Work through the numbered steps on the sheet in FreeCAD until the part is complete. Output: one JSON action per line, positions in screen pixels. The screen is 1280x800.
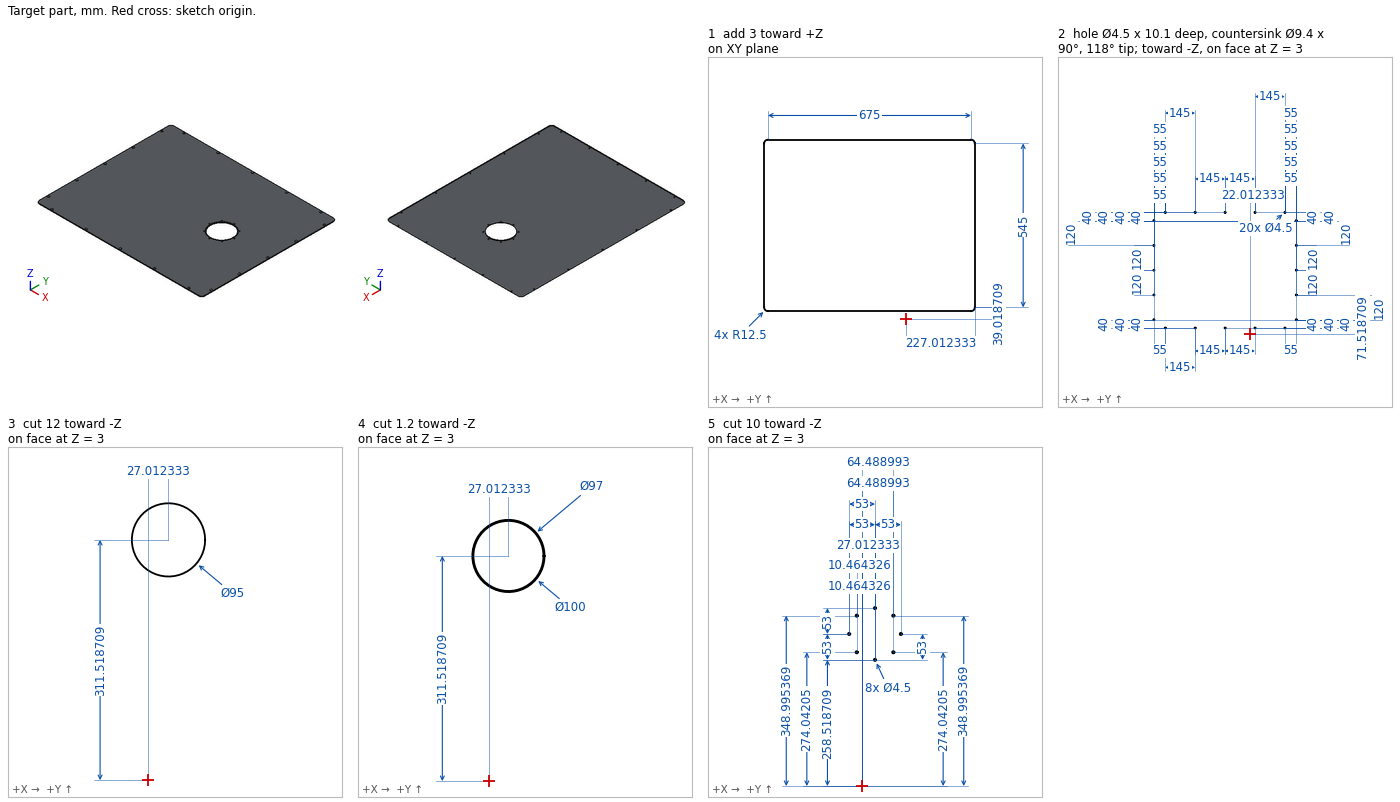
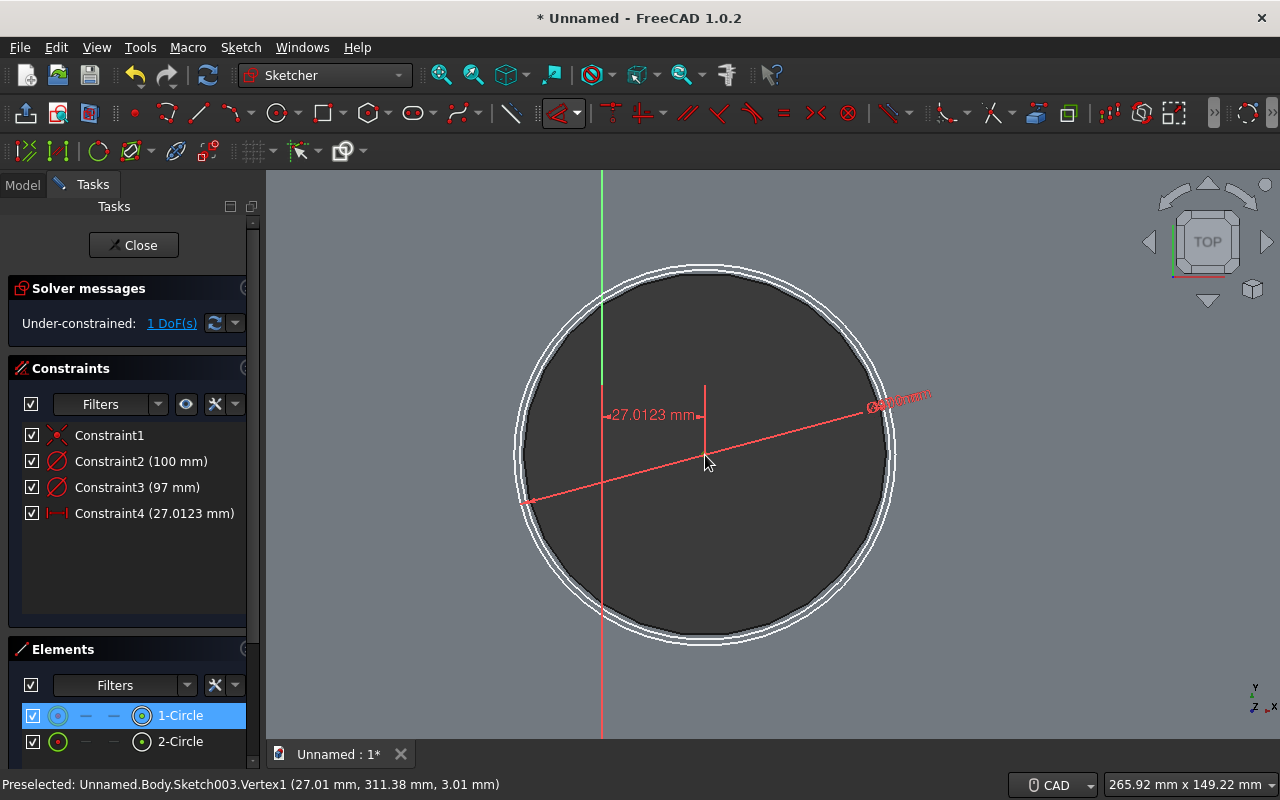
{"action": "left_click", "coordinate": [580, 114]}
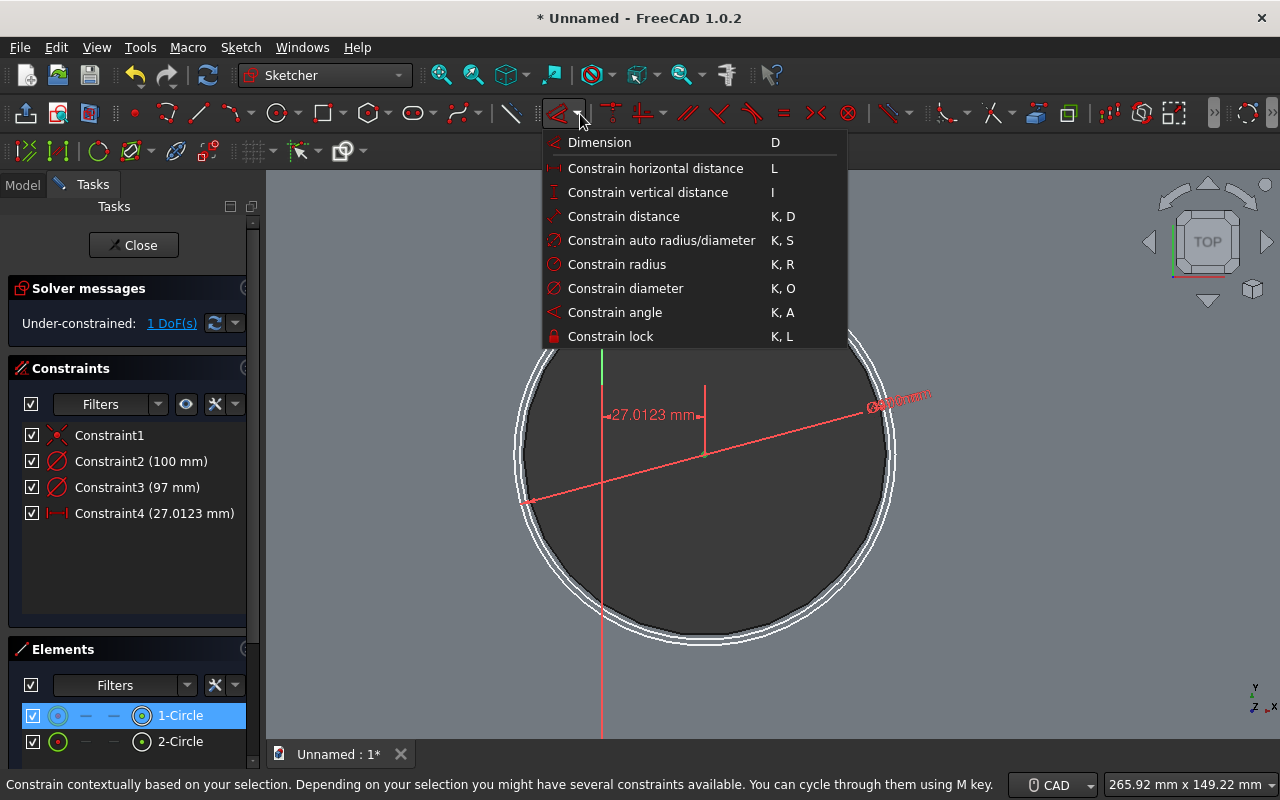
{"action": "left_click", "coordinate": [695, 192]}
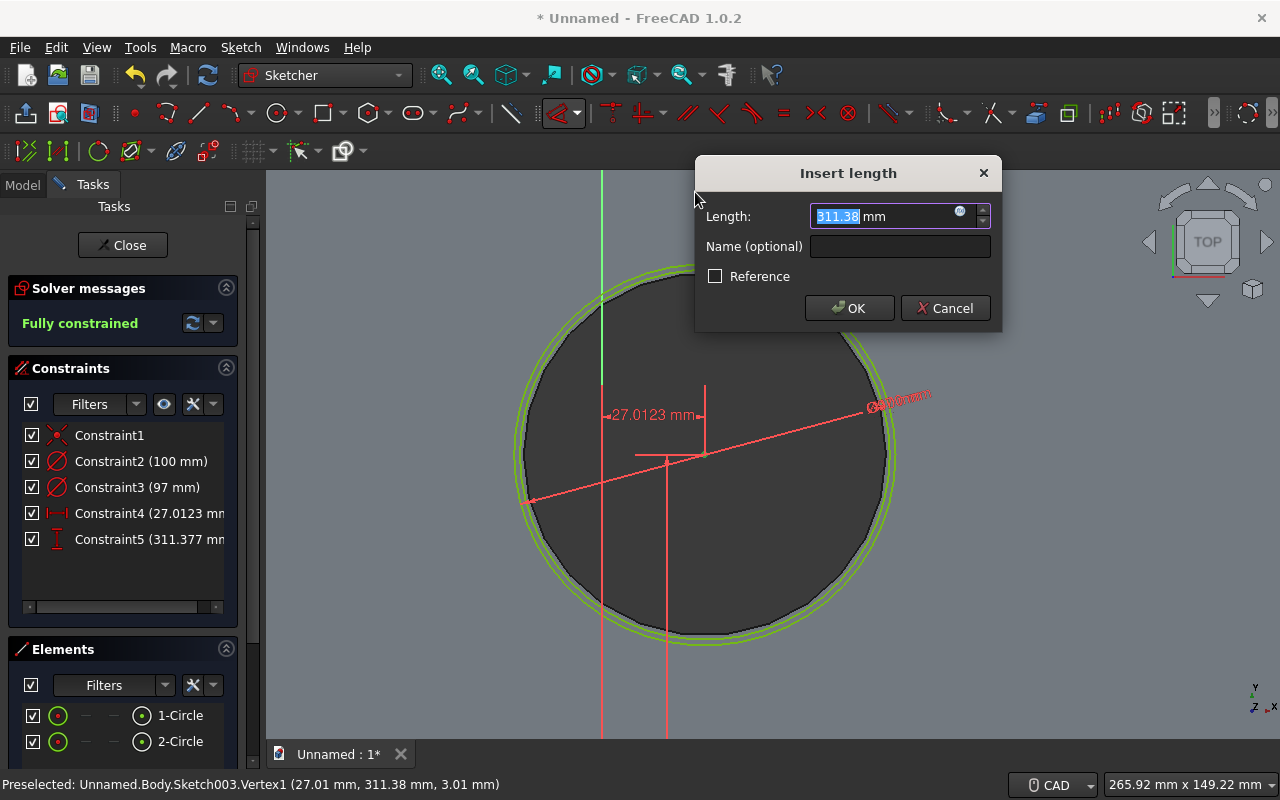
{"action": "type", "text": "311.518709"}
{"action": "key", "text": "Return"}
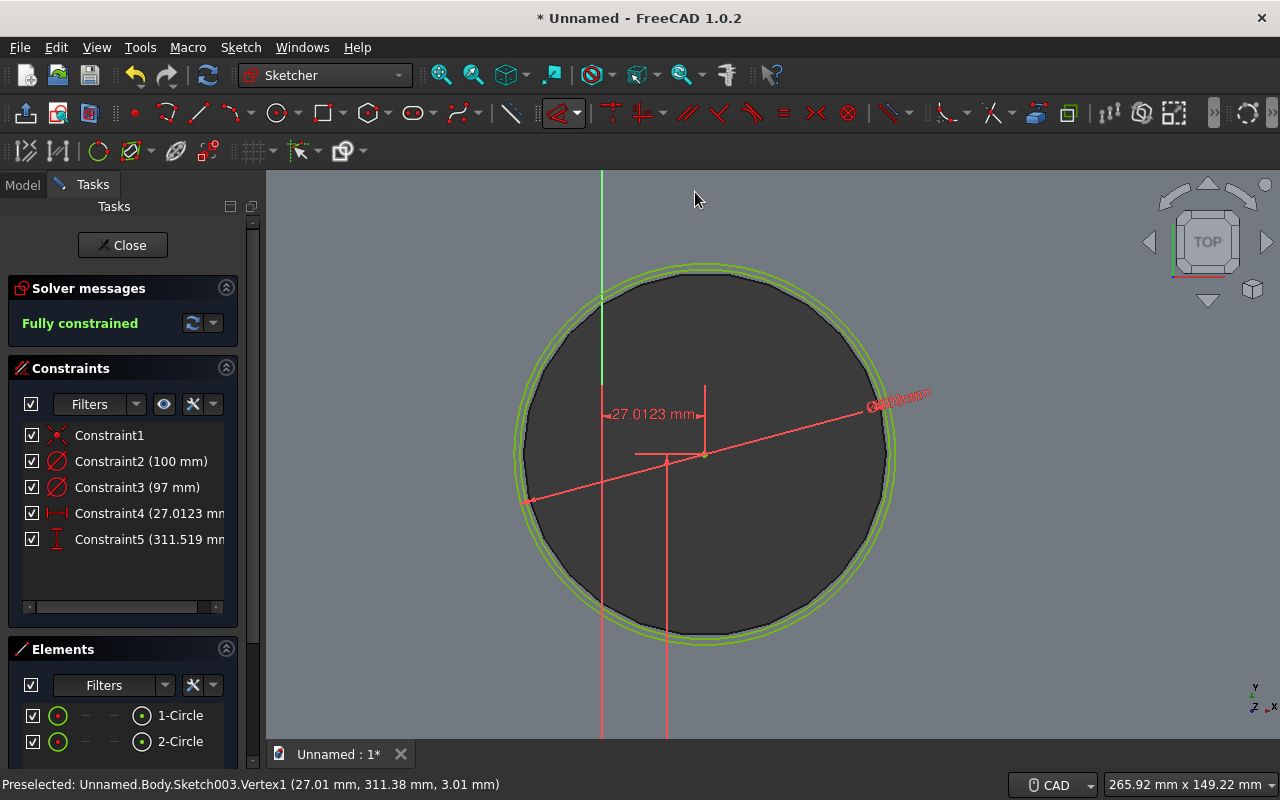
{"action": "left_click", "coordinate": [123, 245]}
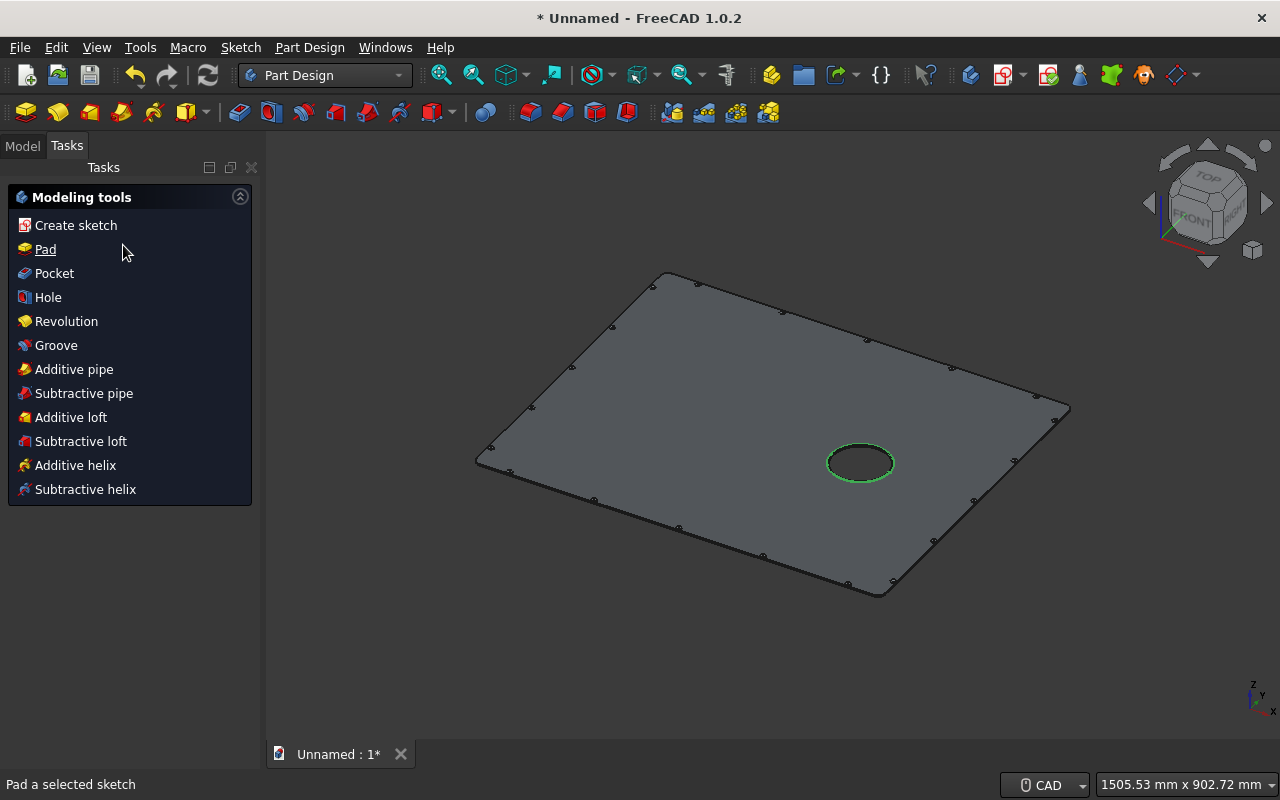
{"action": "left_click", "coordinate": [240, 112]}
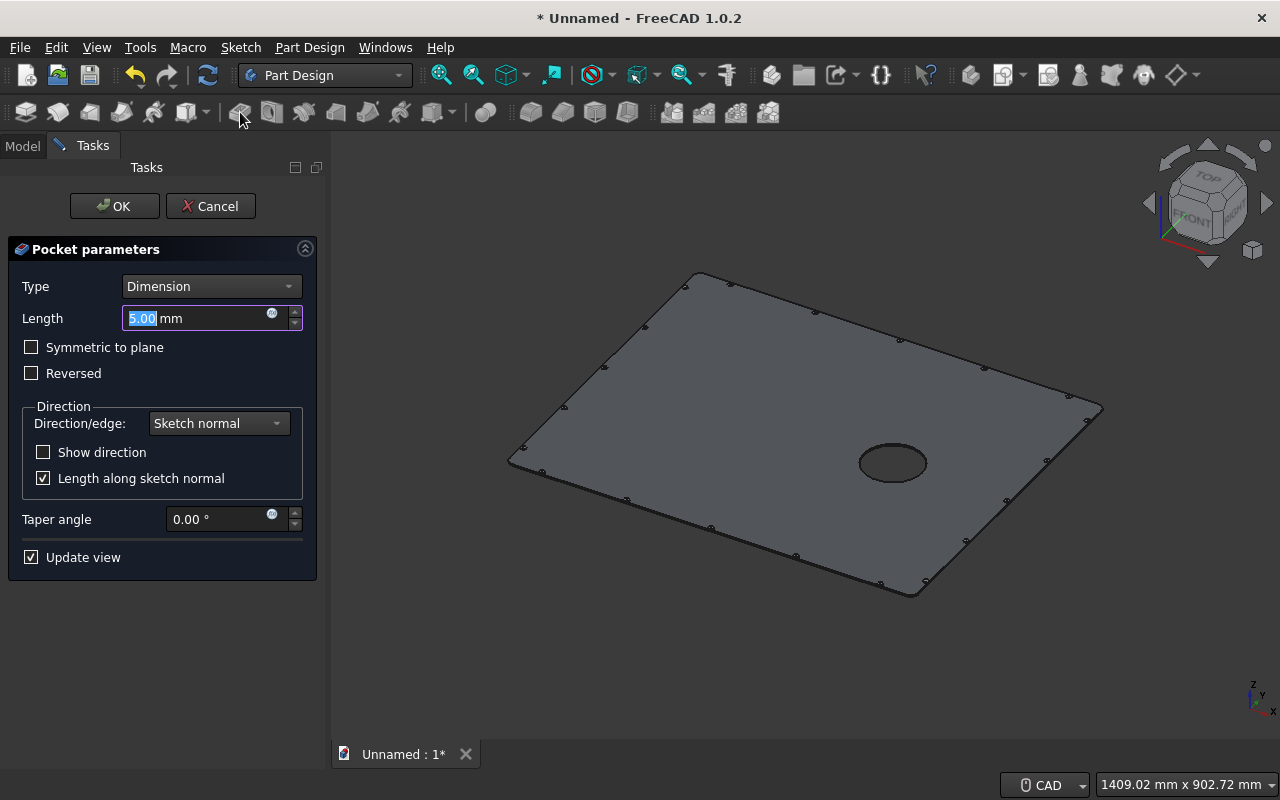
{"action": "type", "text": "1.2"}
{"action": "key", "text": "Tab"}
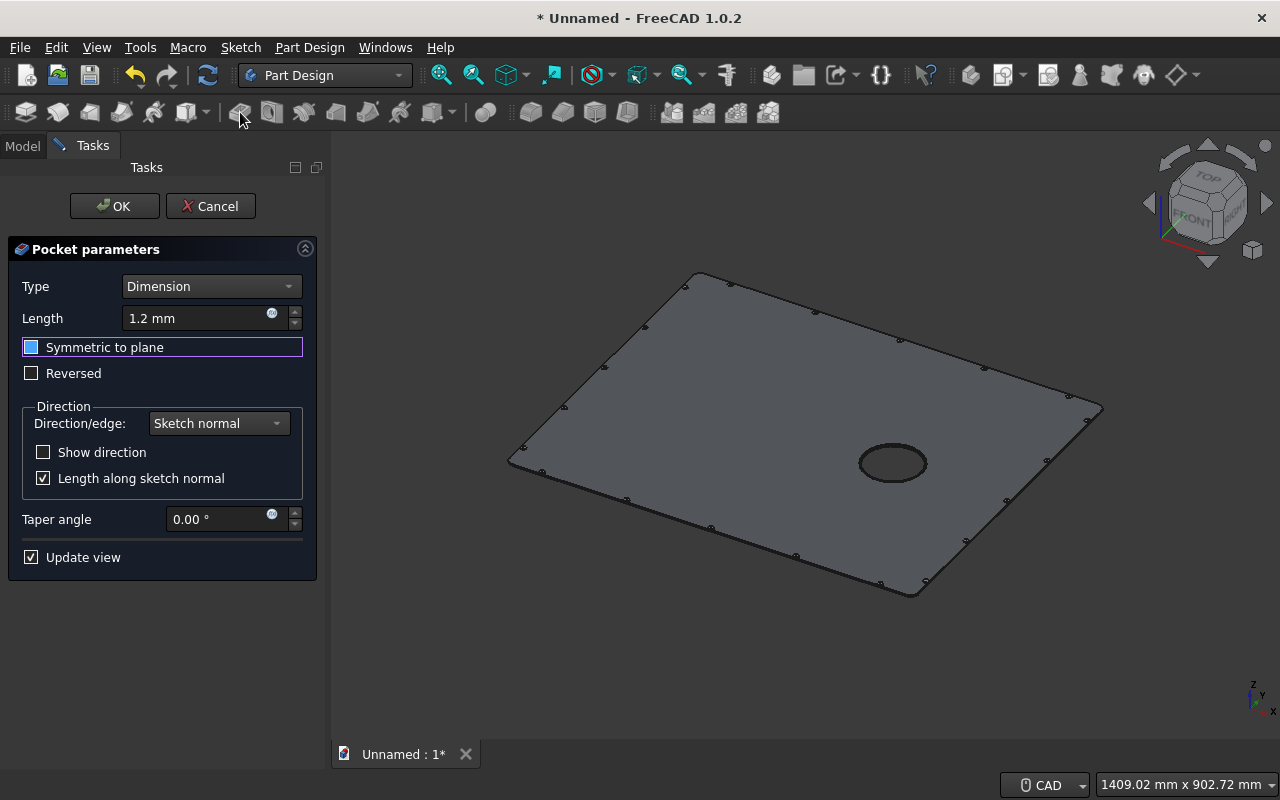
{"action": "left_click", "coordinate": [115, 206]}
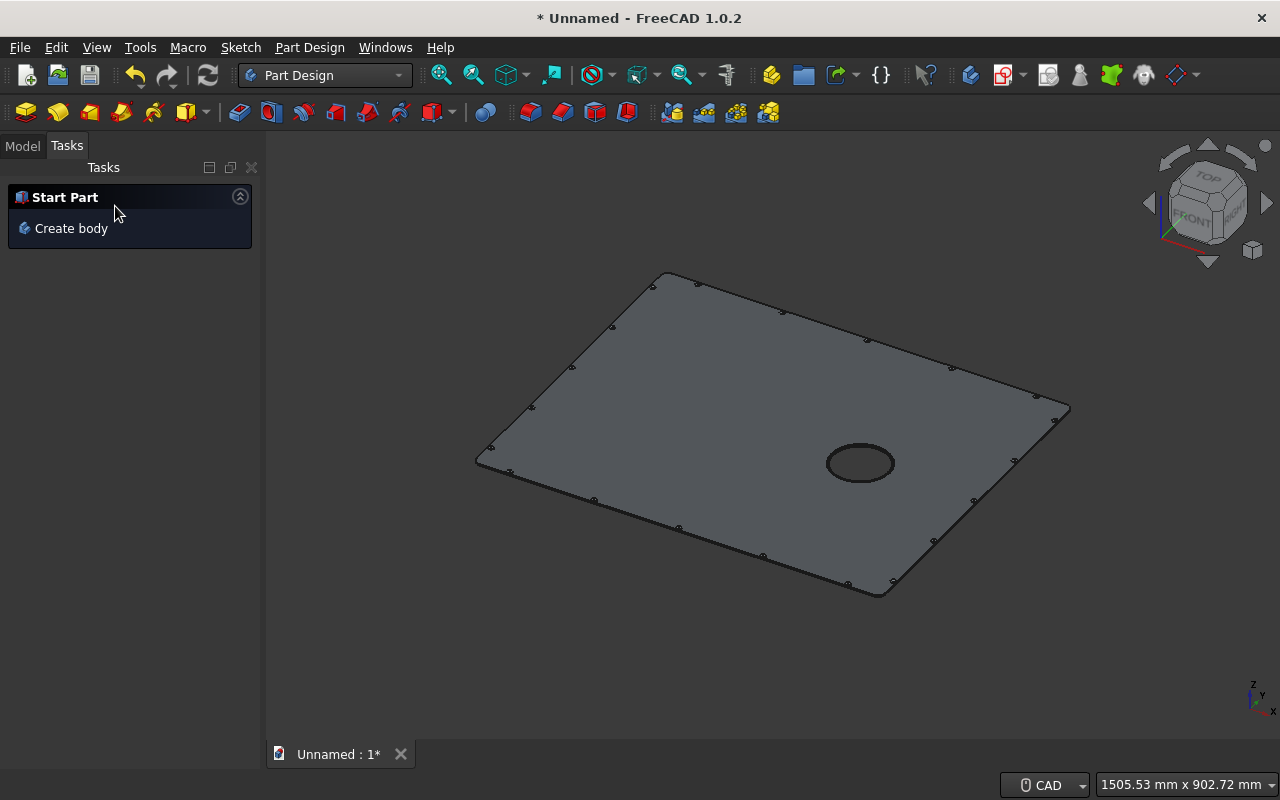
{"action": "left_click", "coordinate": [715, 414]}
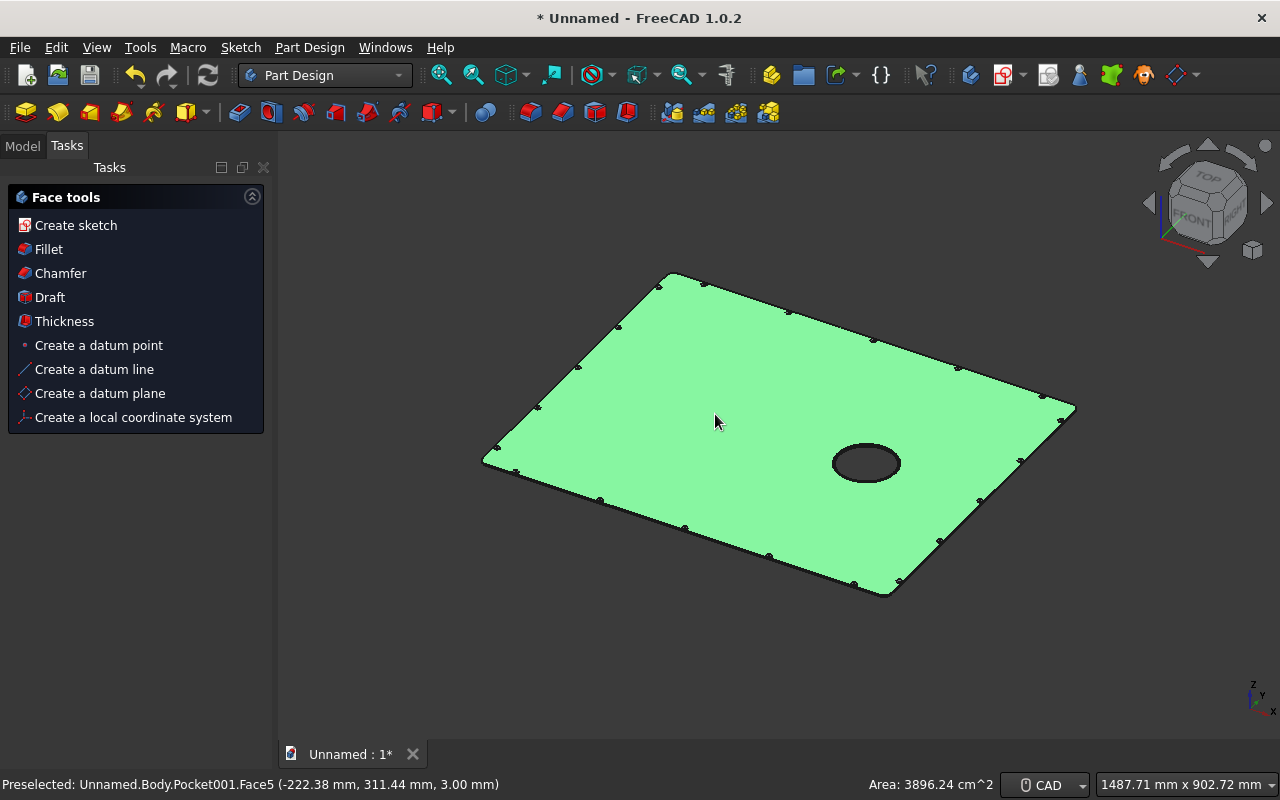
{"action": "left_click", "coordinate": [1004, 76]}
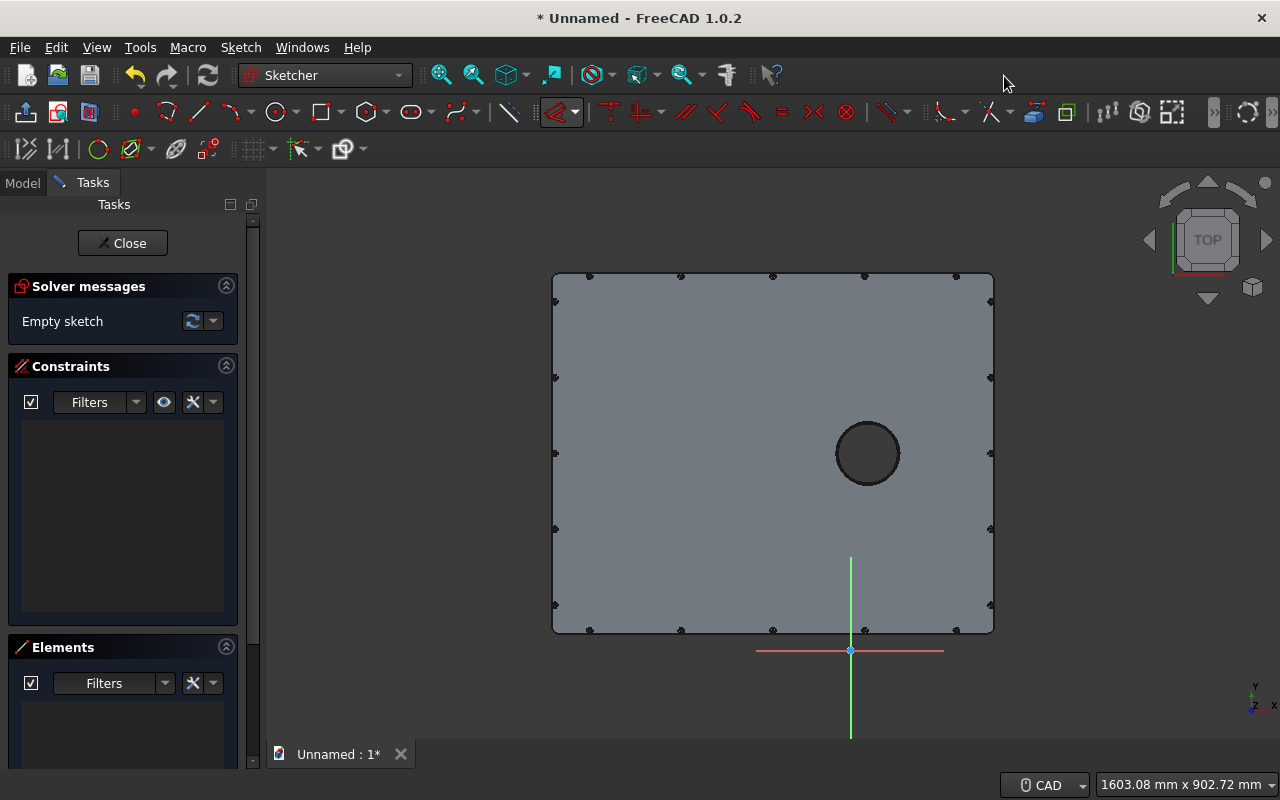
{"action": "scroll", "coordinate": [909, 454], "scroll_direction": "up", "scroll_amount": 8}